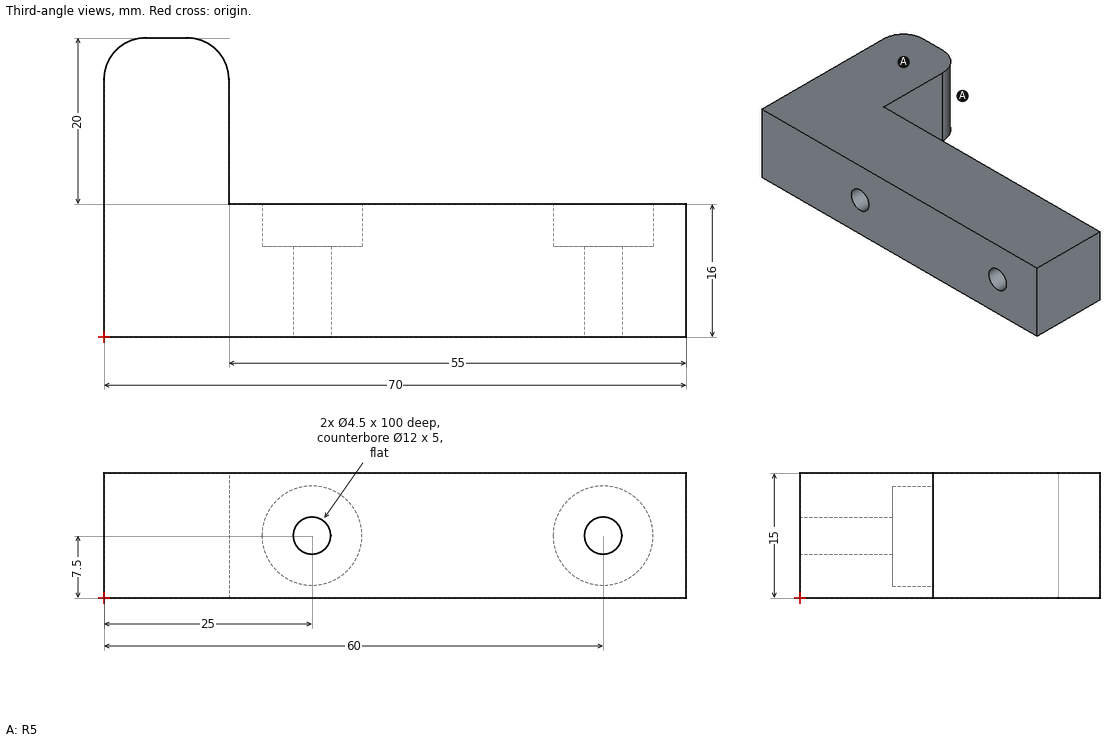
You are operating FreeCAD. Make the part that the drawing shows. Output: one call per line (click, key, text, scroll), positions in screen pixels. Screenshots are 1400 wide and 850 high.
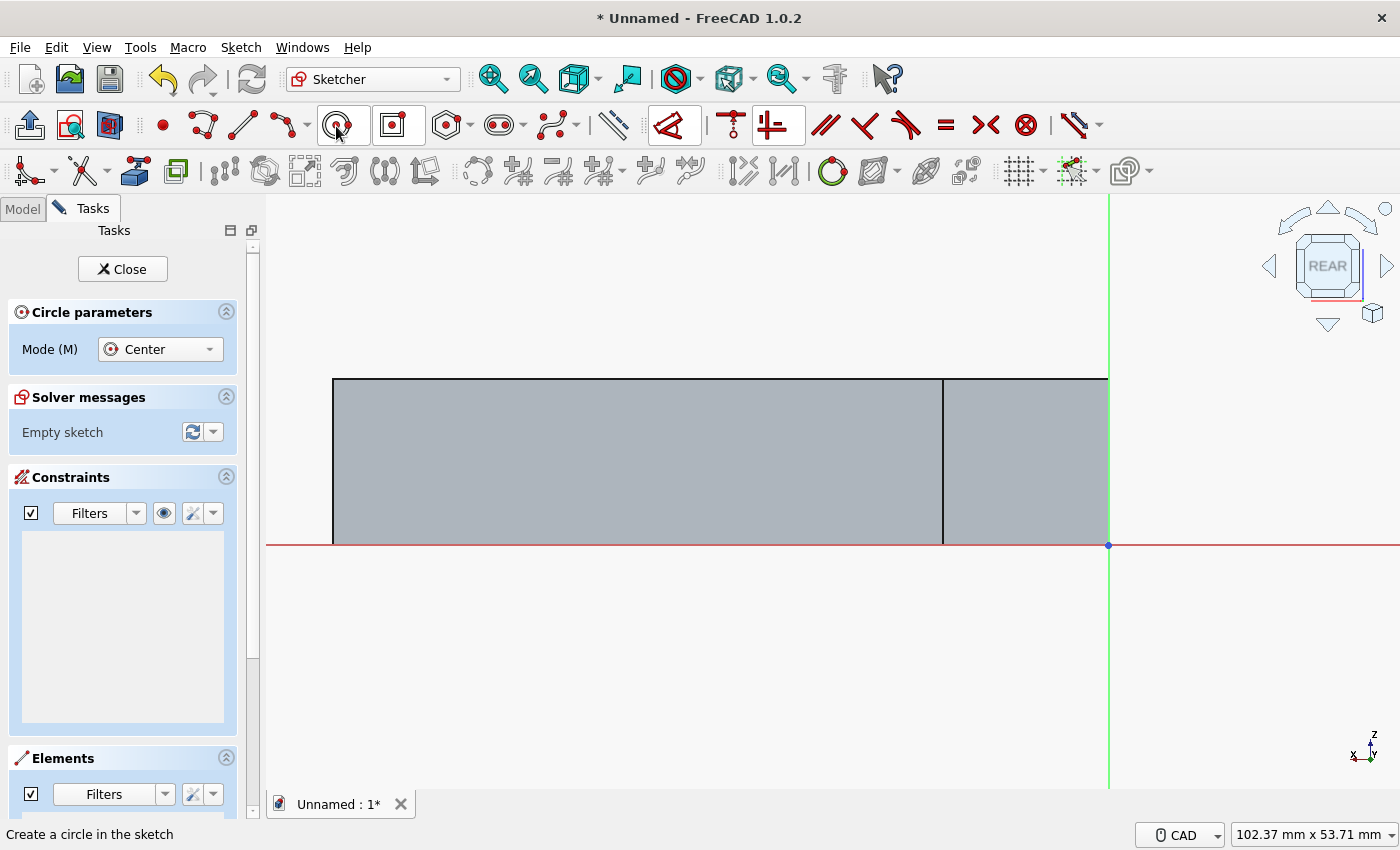
click(832, 462)
move(849, 444)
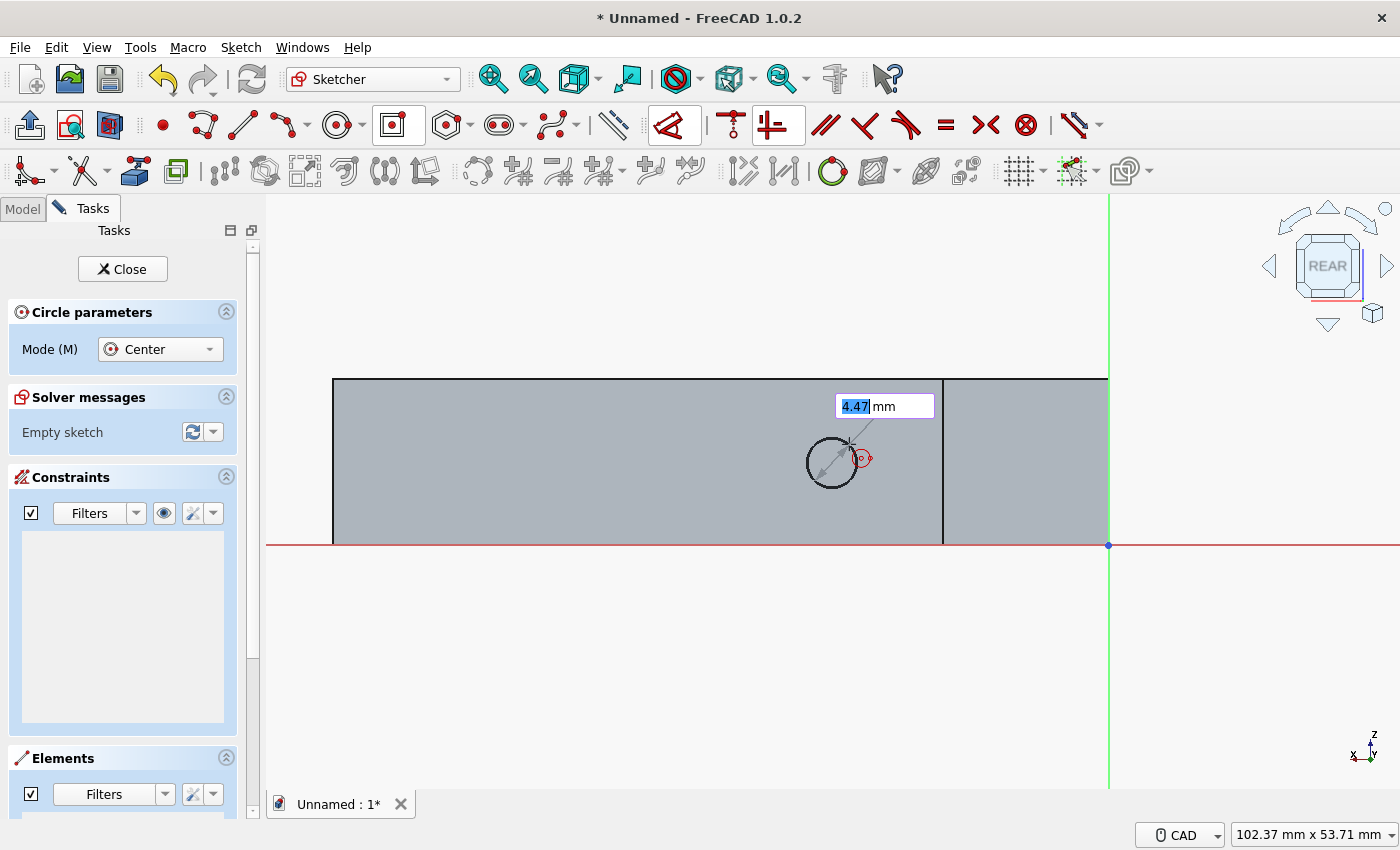
text(4.5)
key(Return)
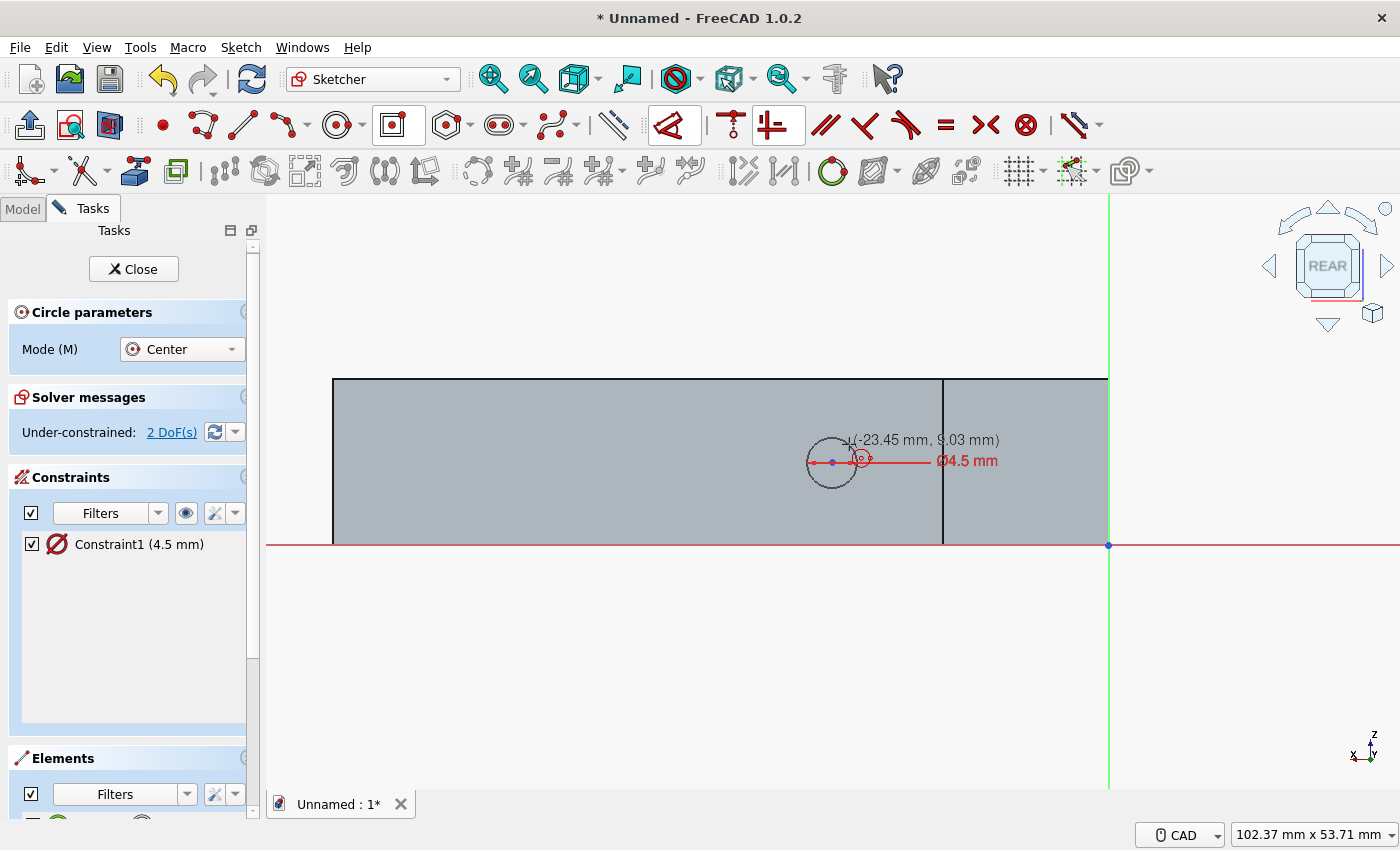
click(444, 462)
move(462, 444)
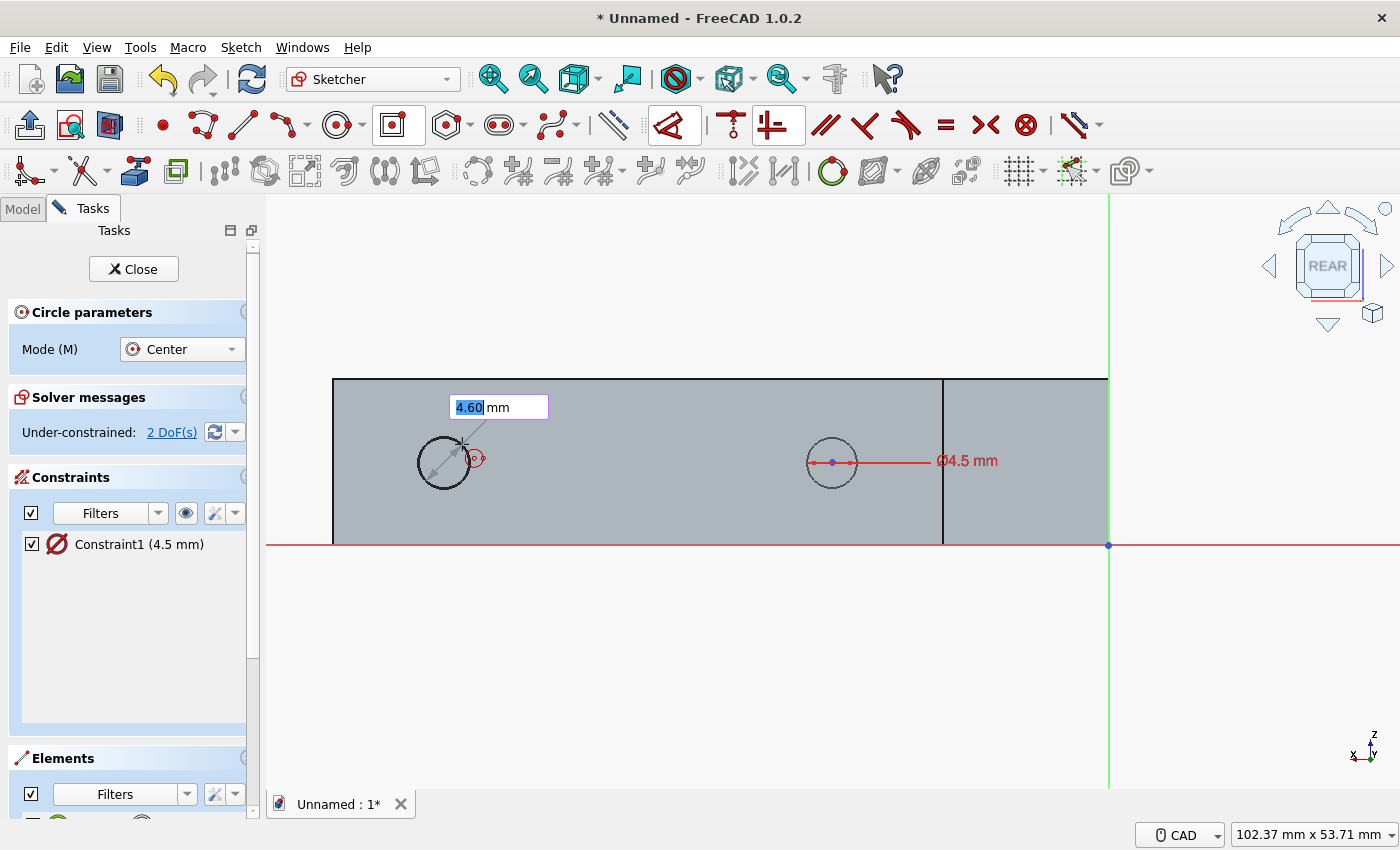
text(4.5)
key(Return)
key(Escape)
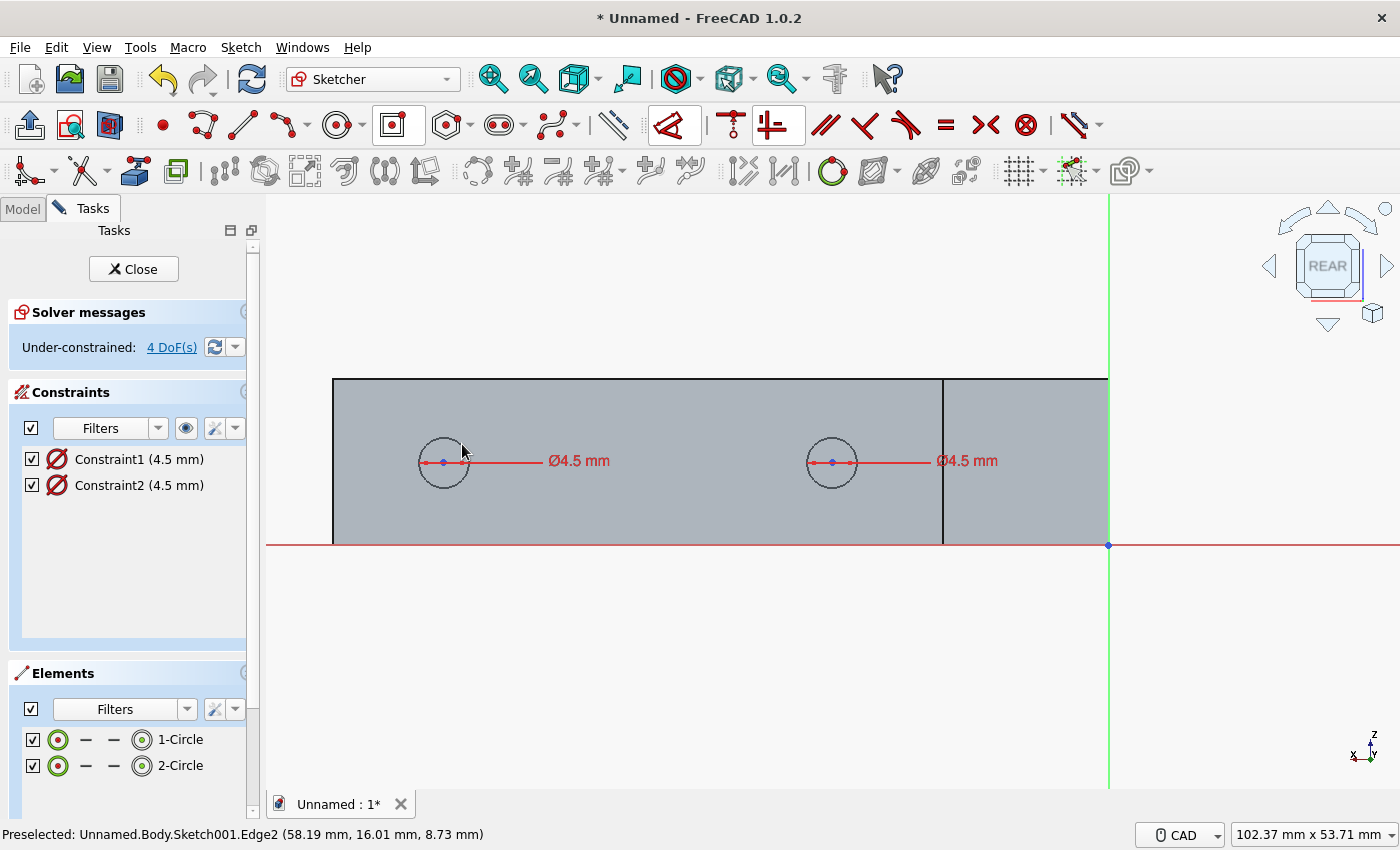
click(832, 463)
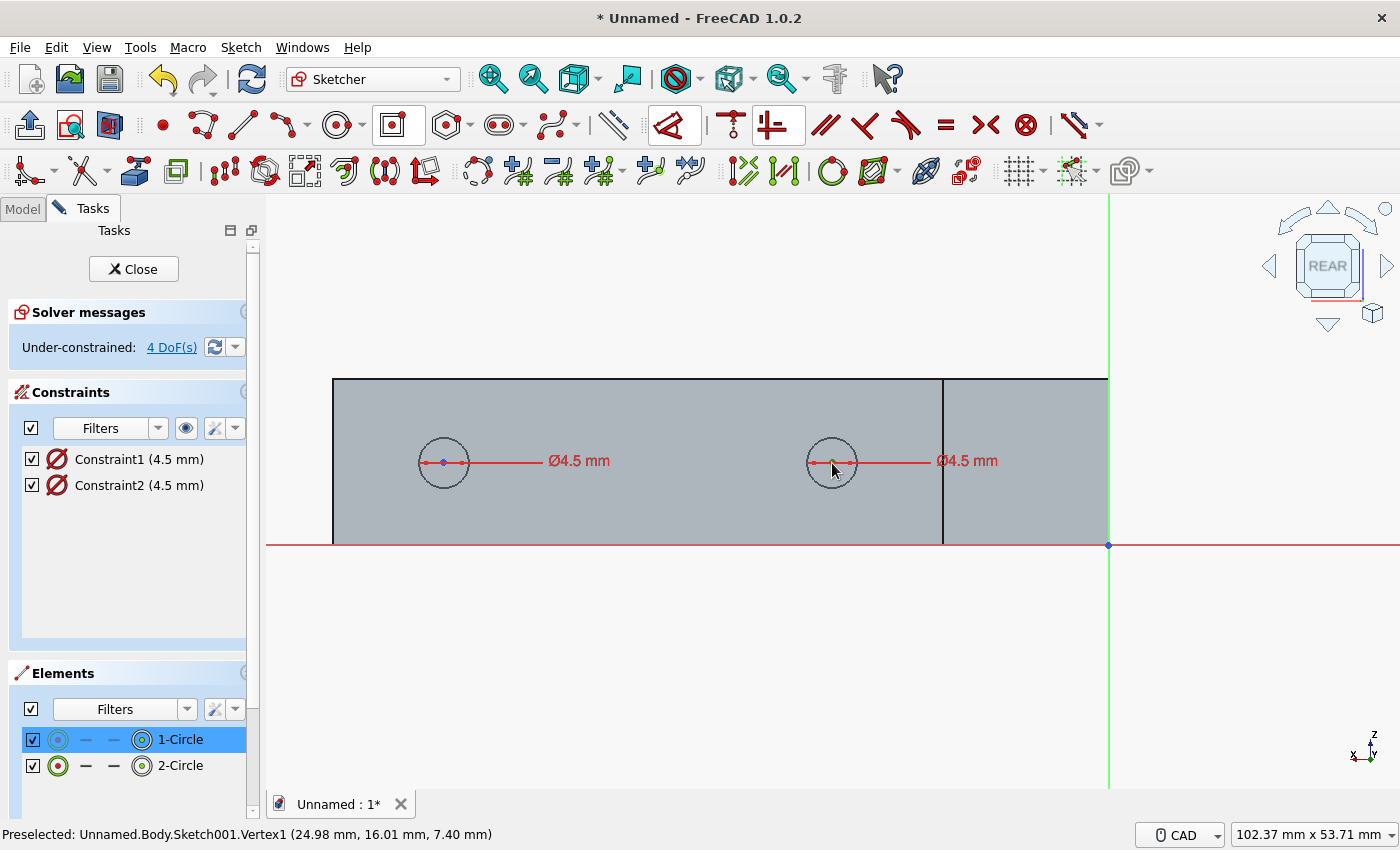
click(444, 463)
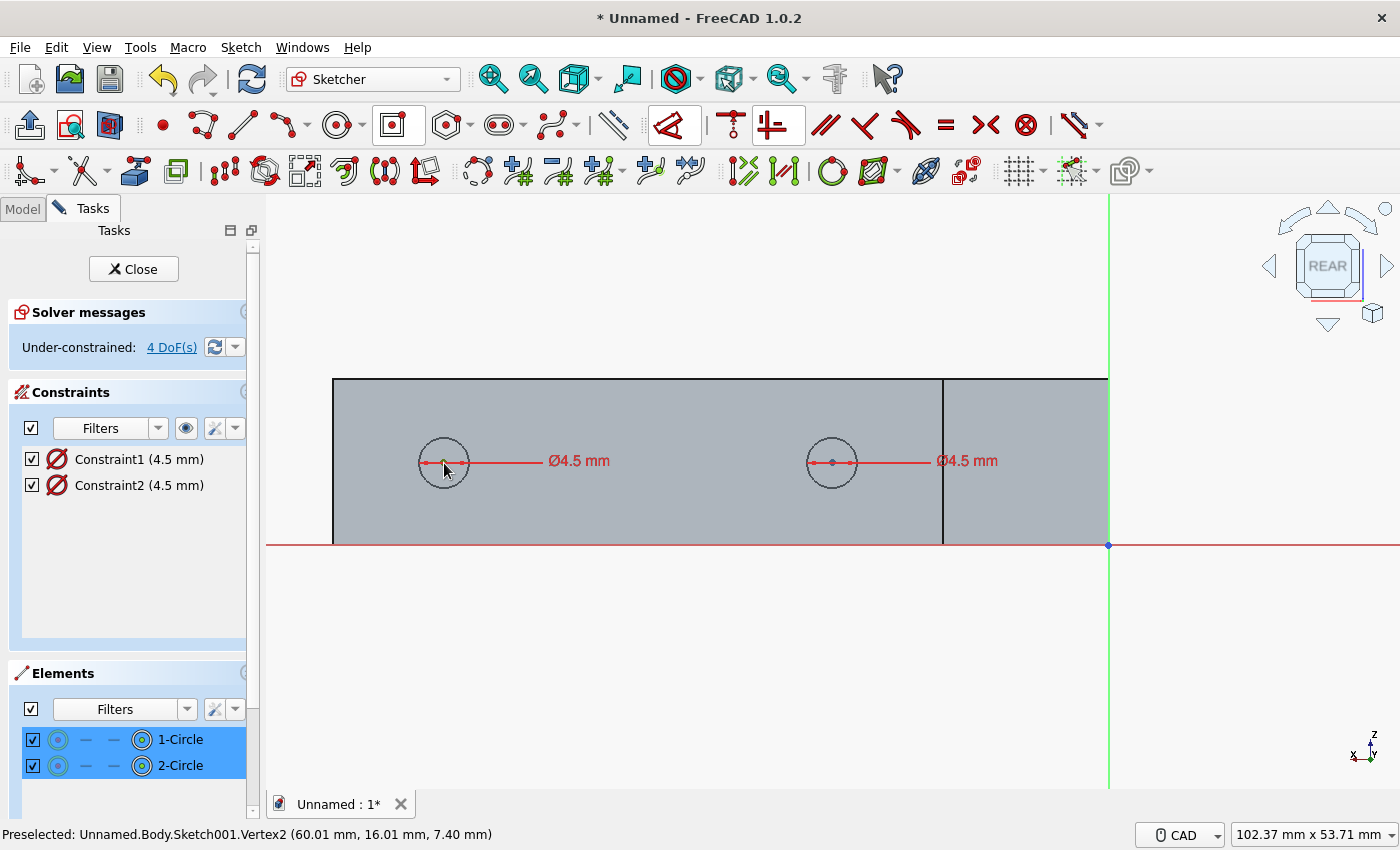
click(800, 126)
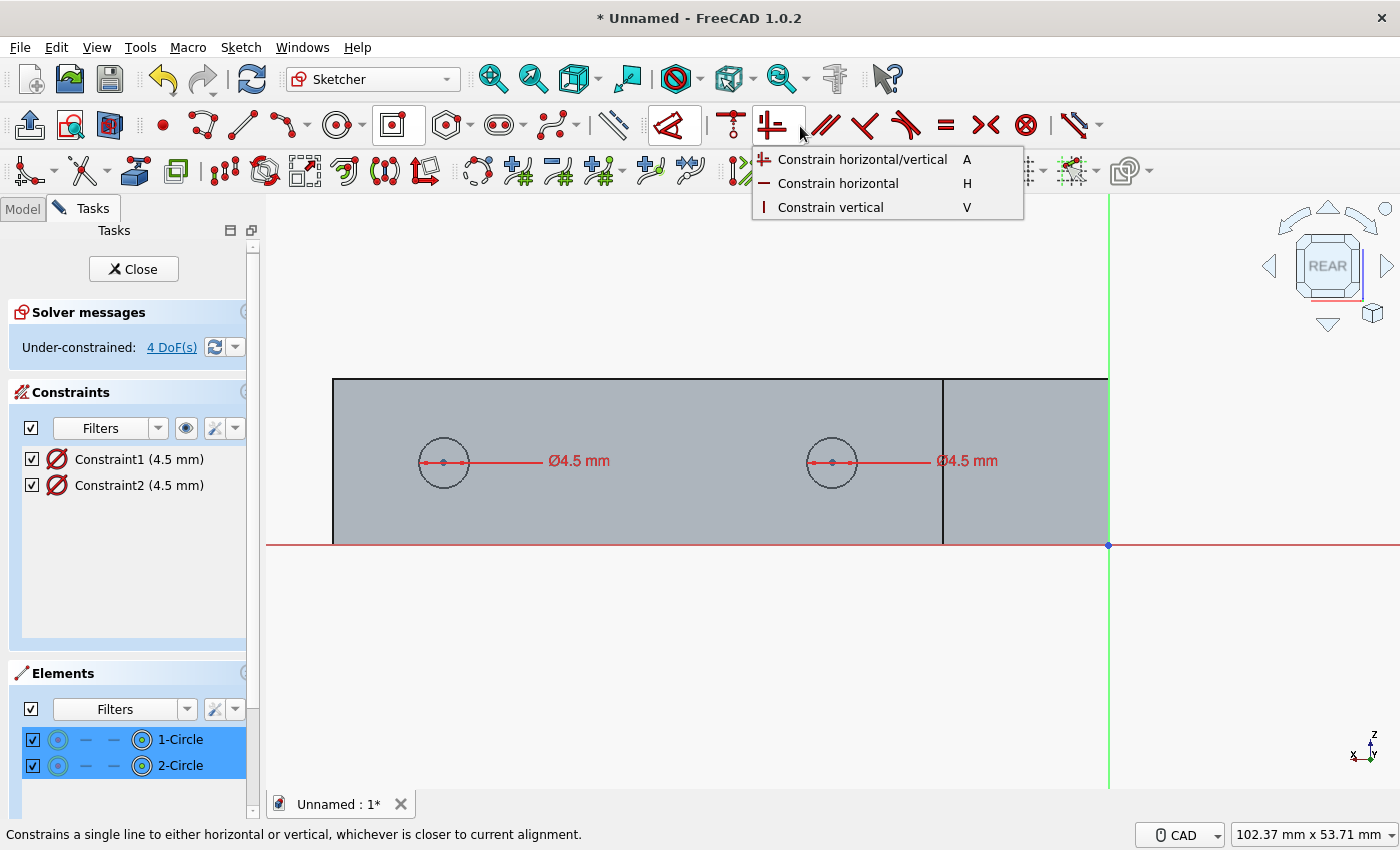
click(888, 183)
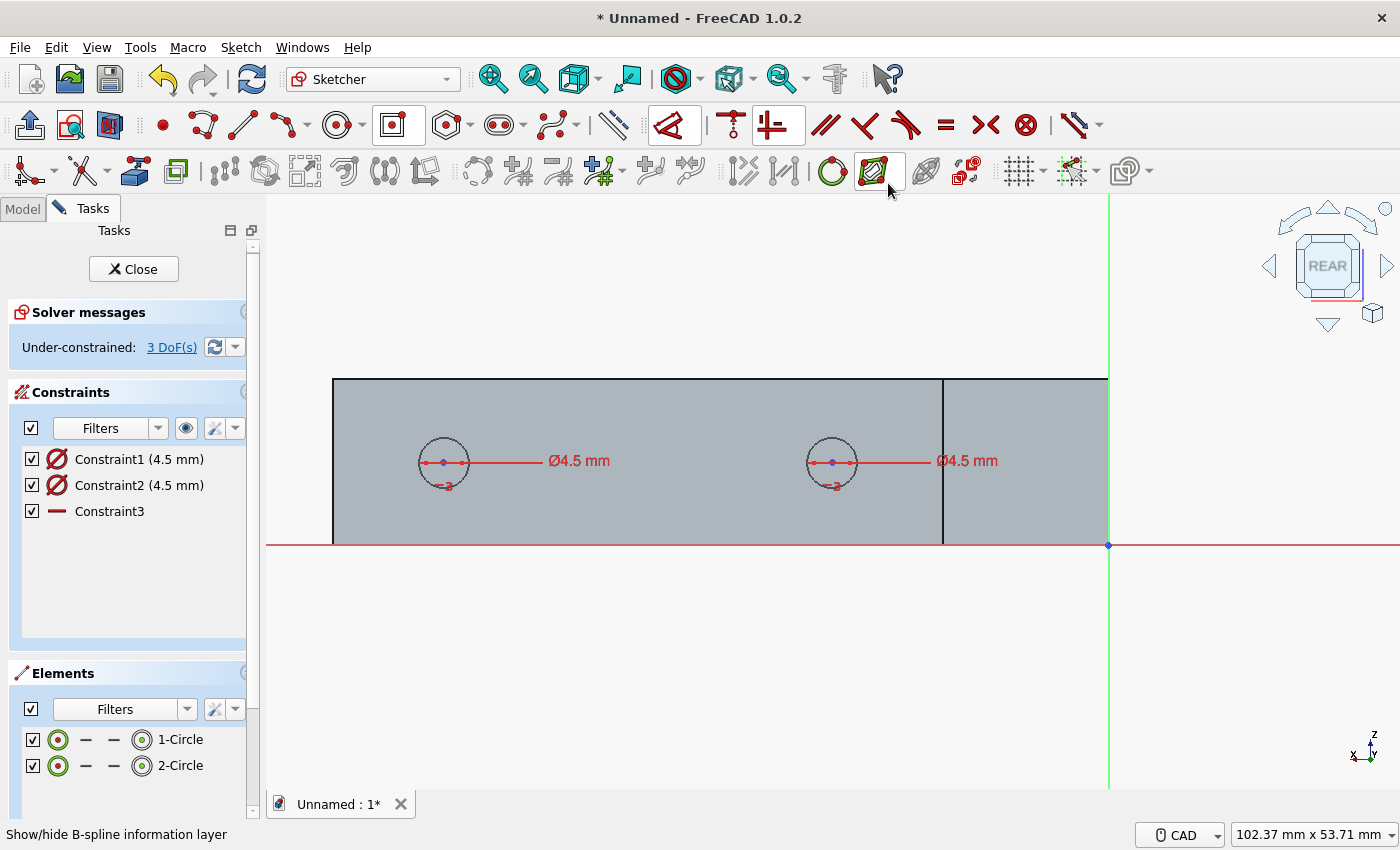
click(832, 463)